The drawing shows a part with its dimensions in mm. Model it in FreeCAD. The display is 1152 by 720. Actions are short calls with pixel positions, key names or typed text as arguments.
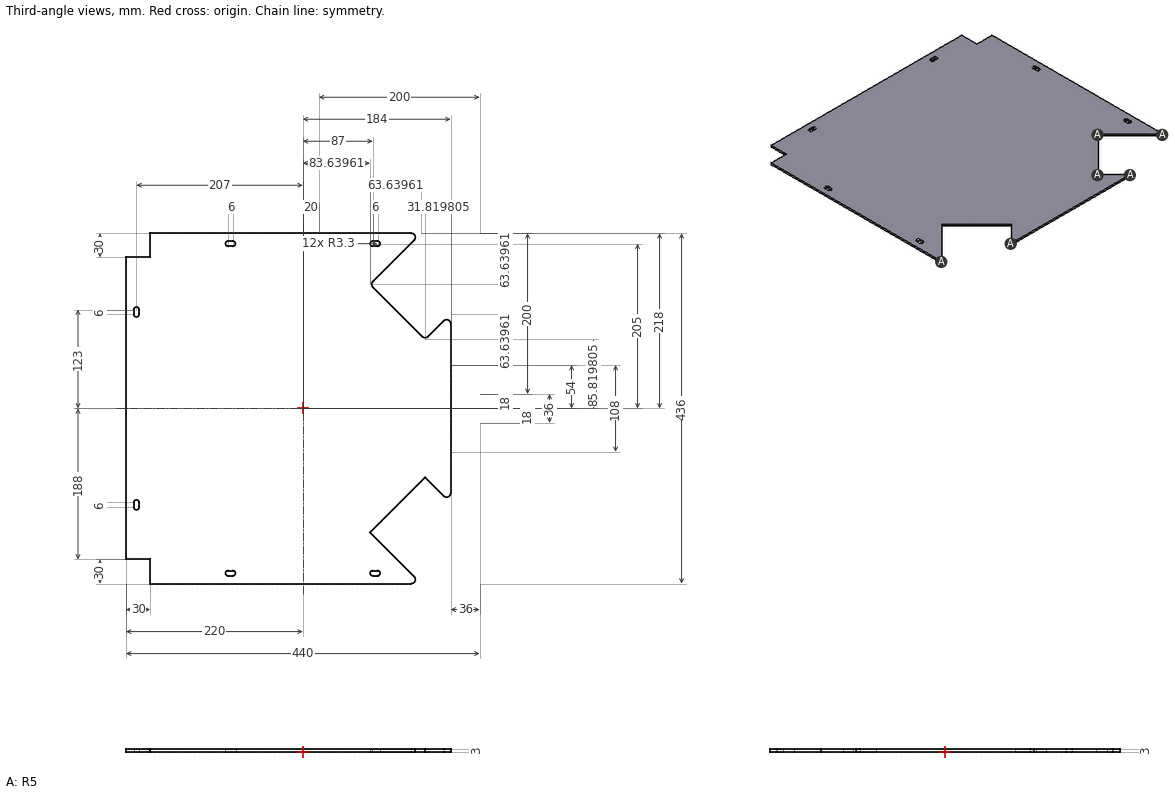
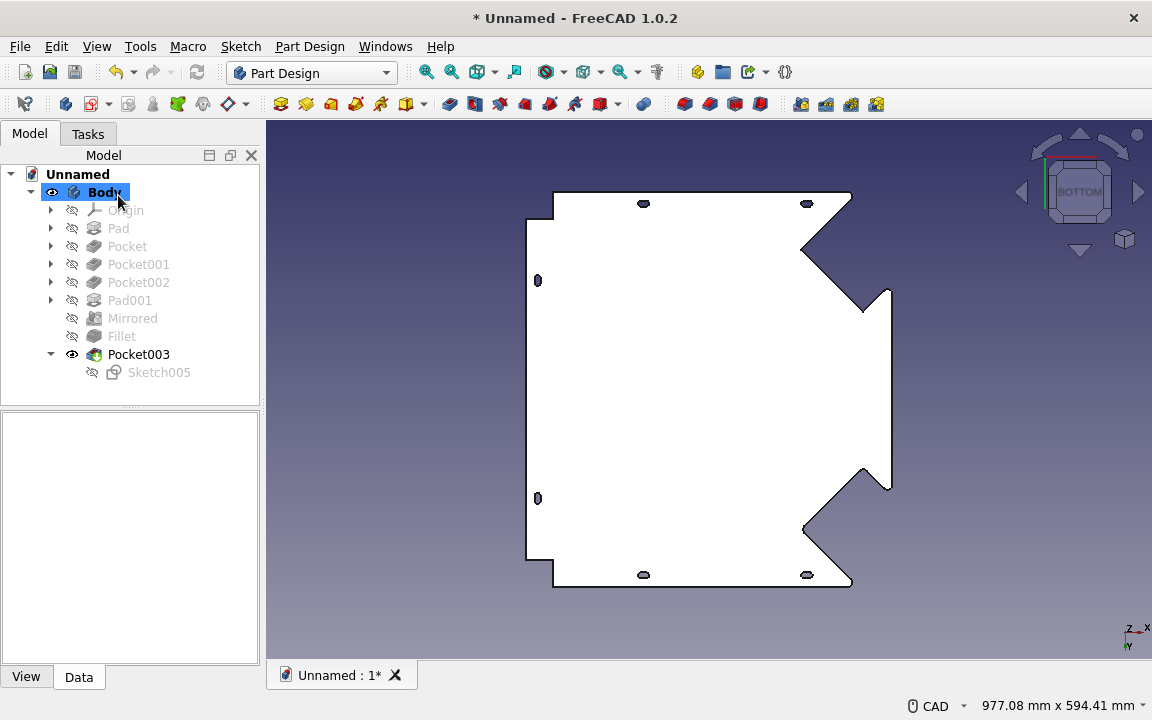
key(0)